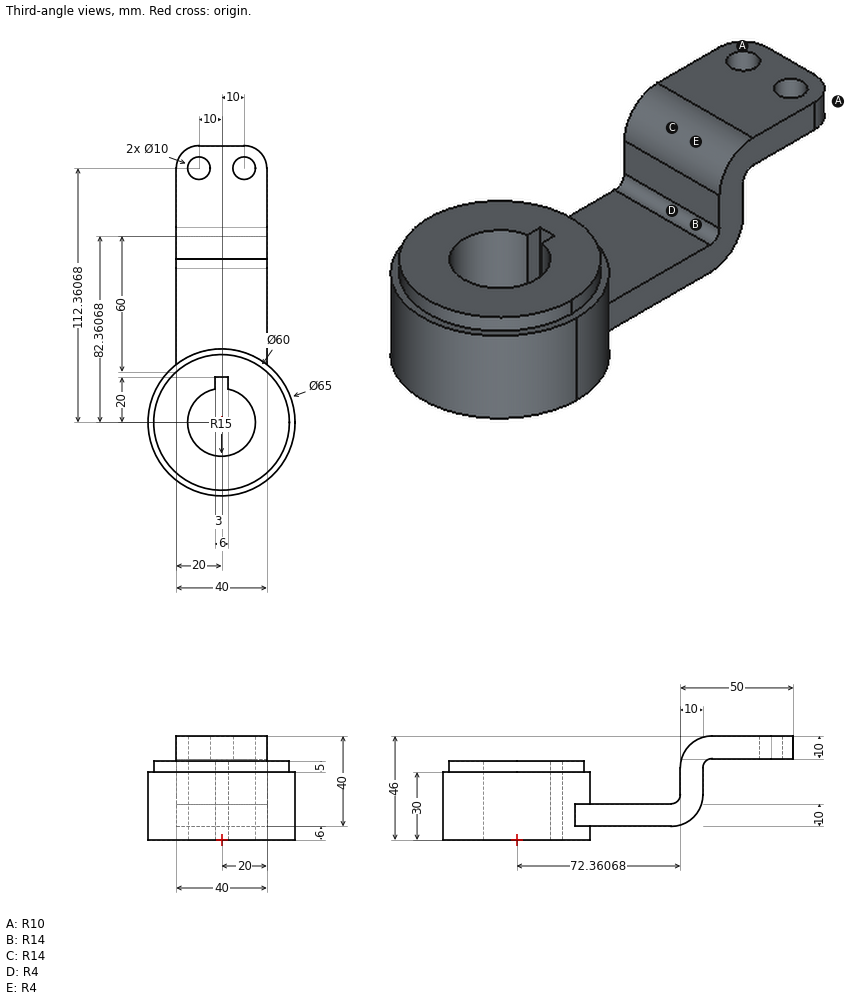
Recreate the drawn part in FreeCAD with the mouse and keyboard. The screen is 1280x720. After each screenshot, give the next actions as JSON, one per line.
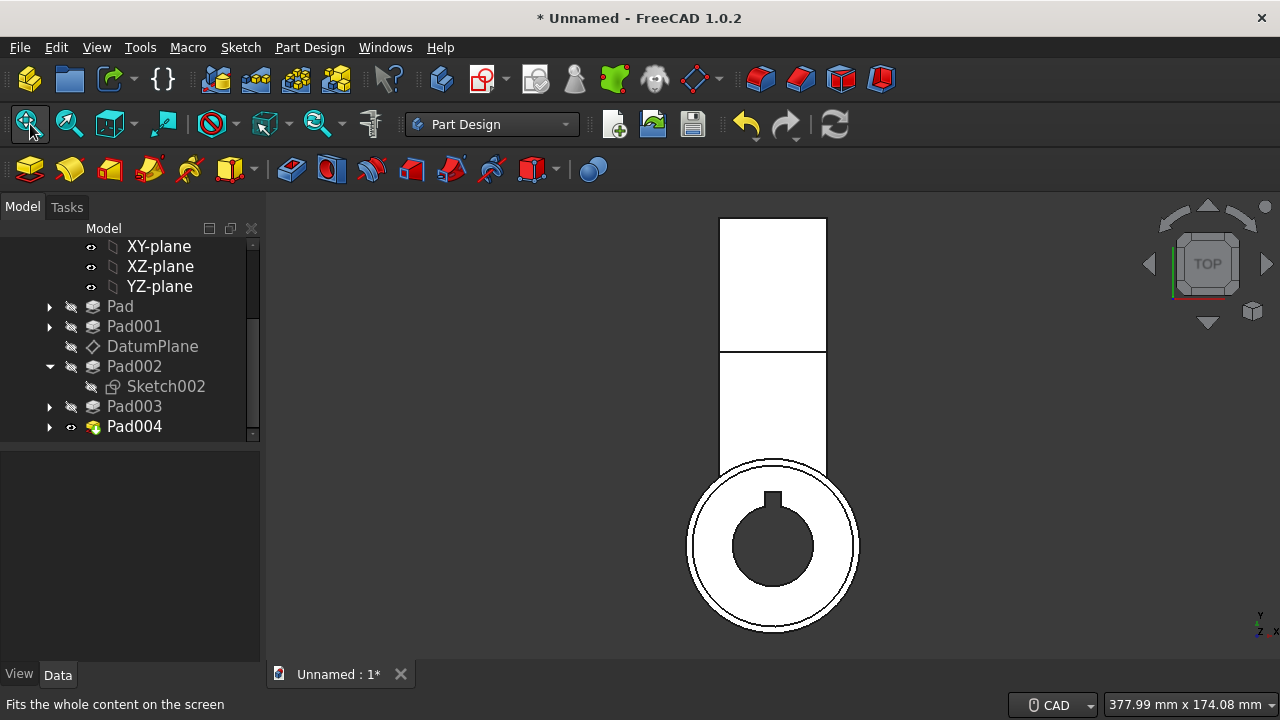
{"action": "key", "text": "0"}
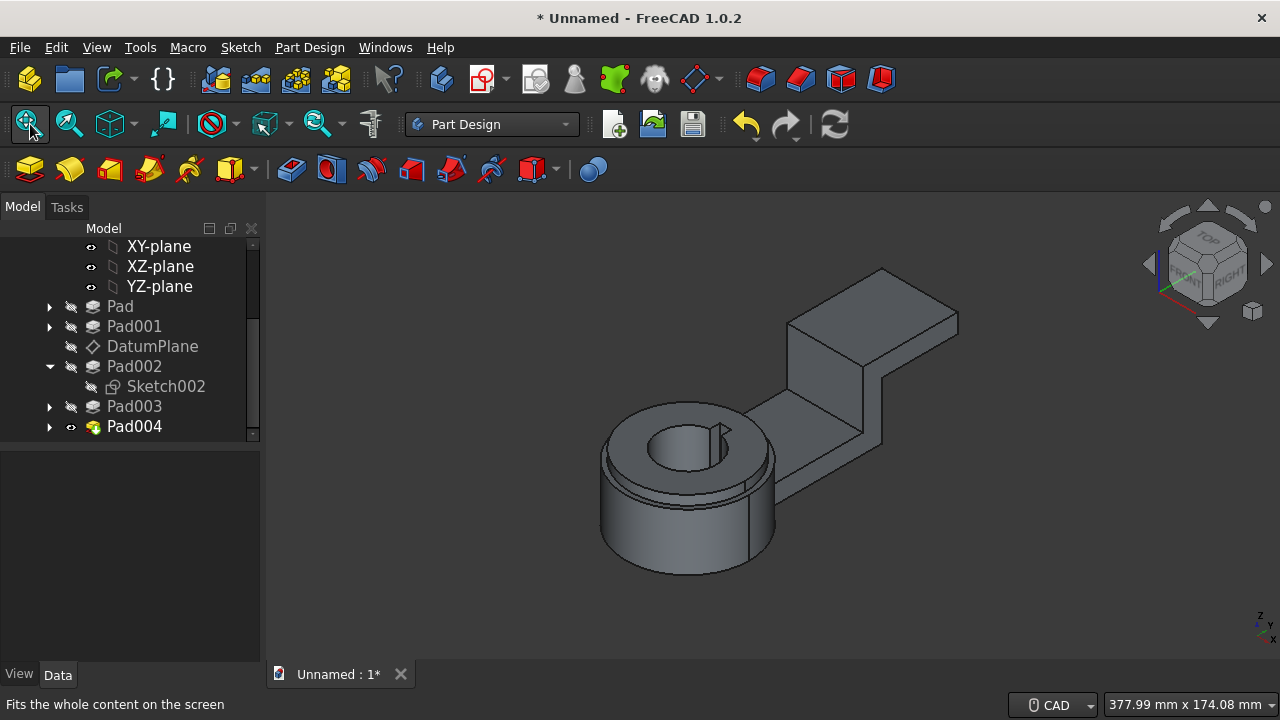
{"action": "key", "text": "1"}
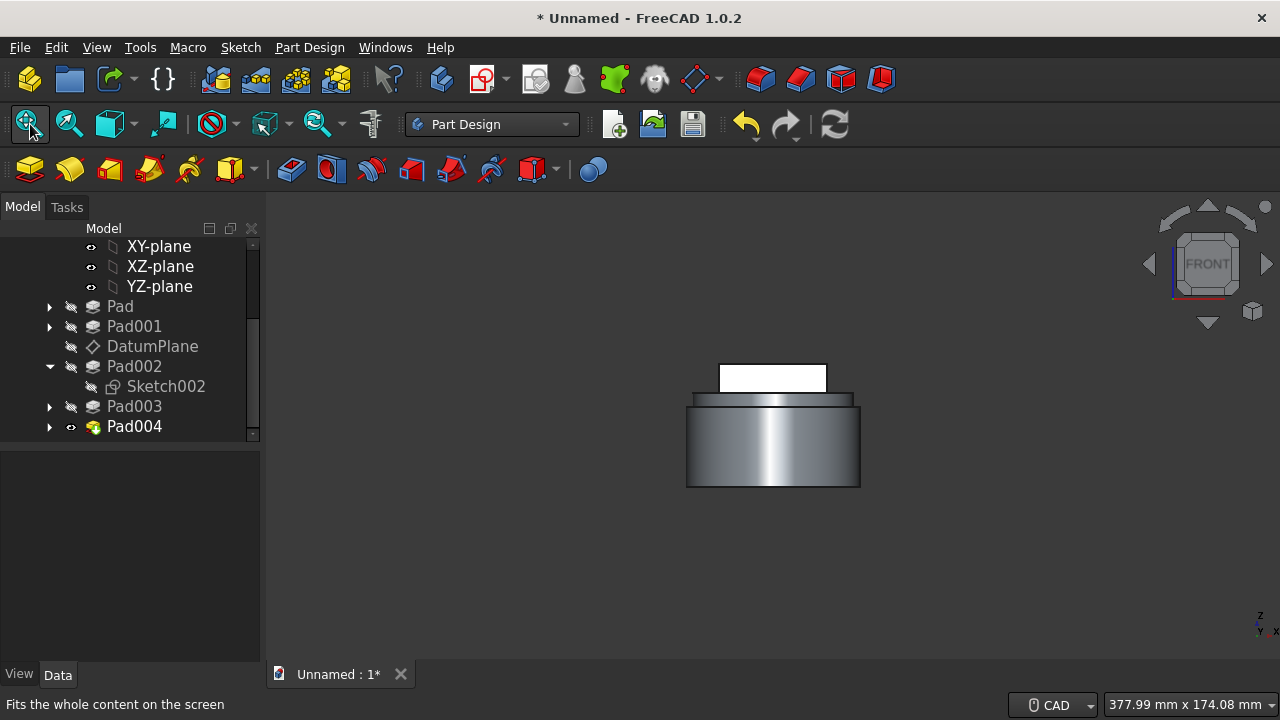
{"action": "key", "text": "v f"}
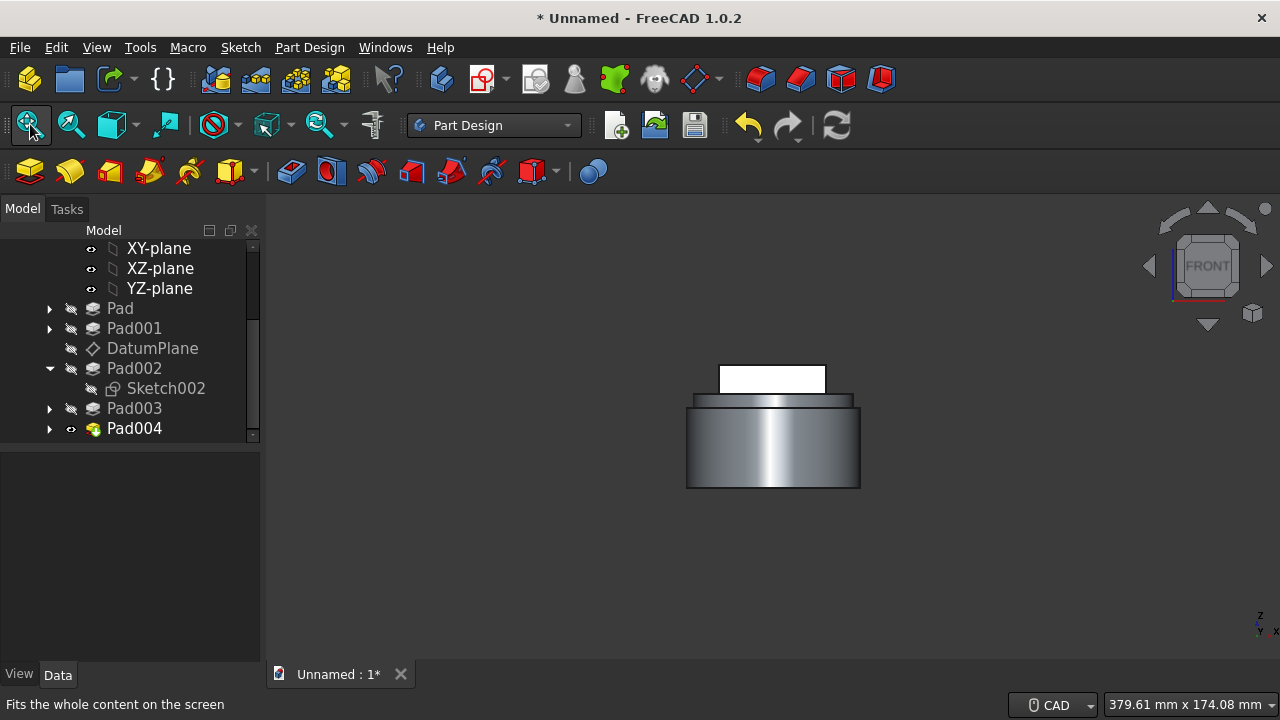
{"action": "key", "text": "3"}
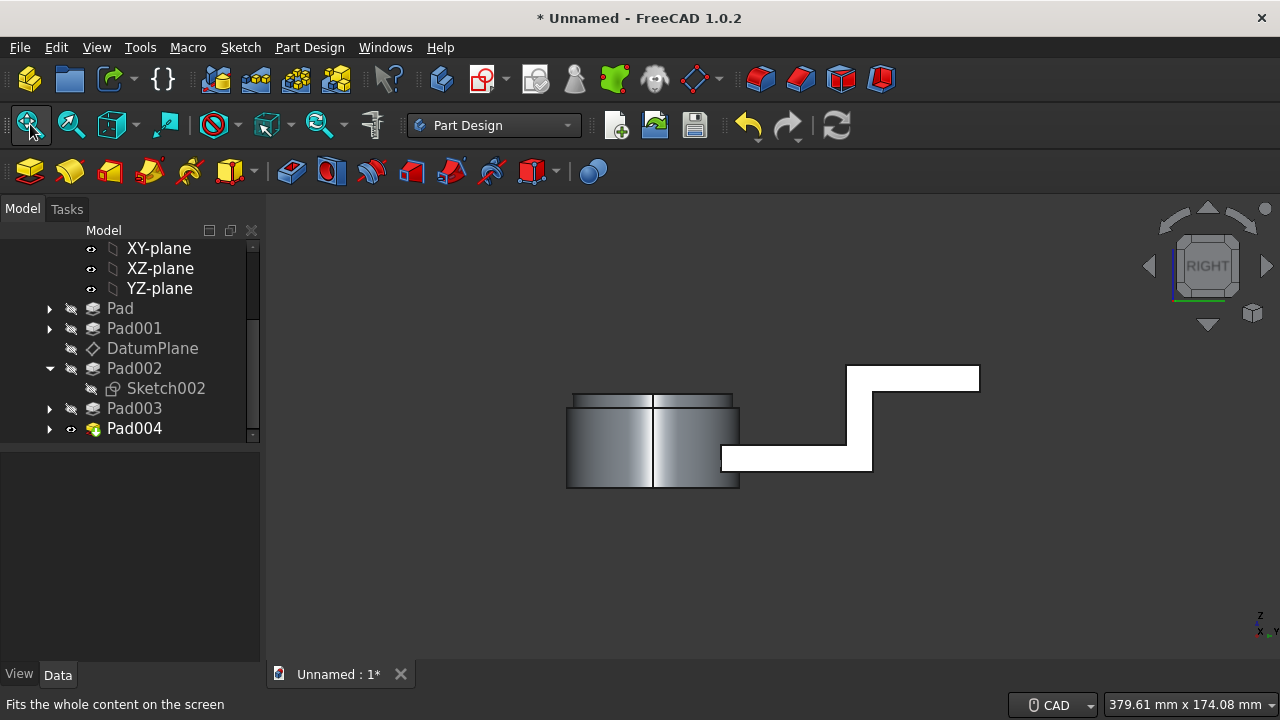
{"action": "key", "text": "v f"}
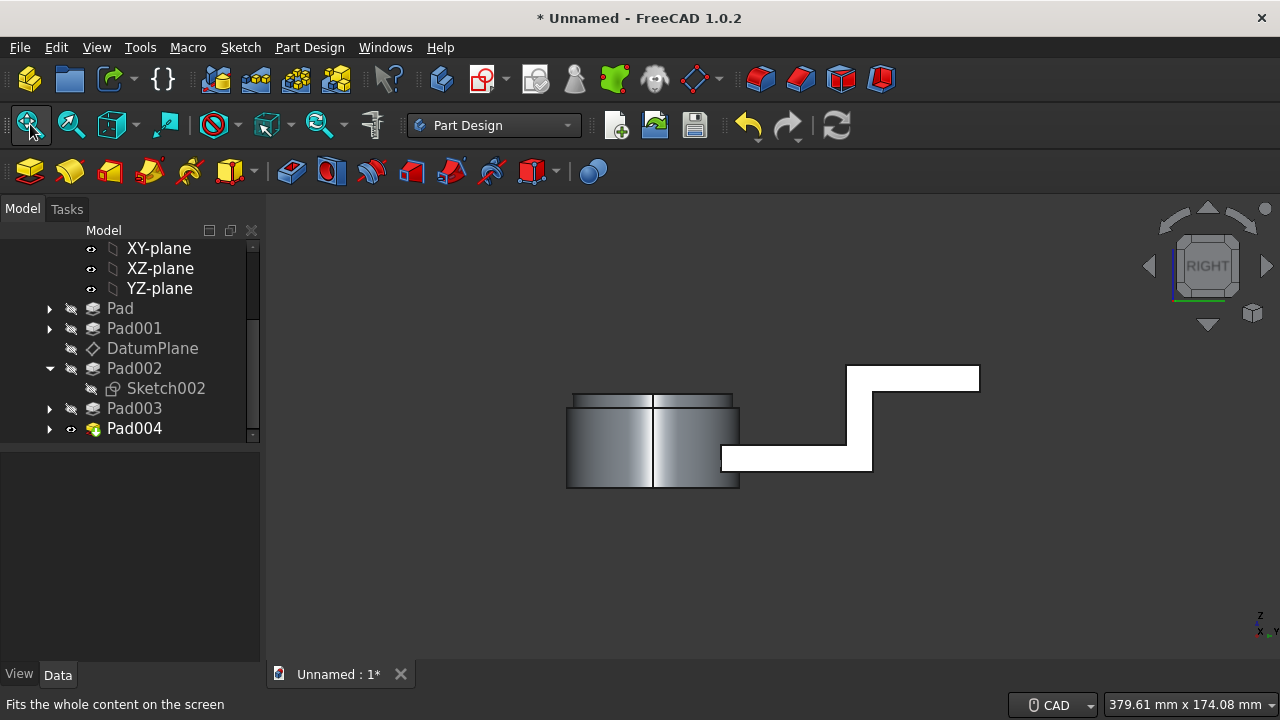
{"action": "left_click", "coordinate": [980, 377]}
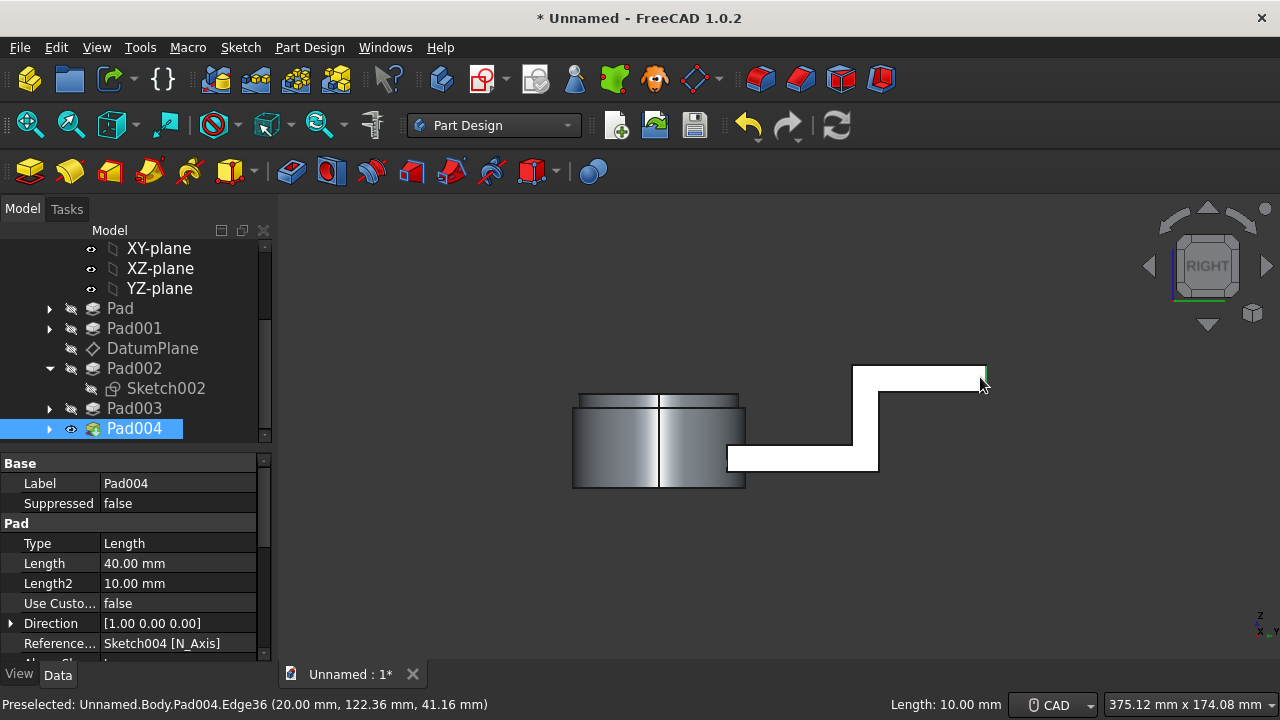
{"action": "key", "text": "5"}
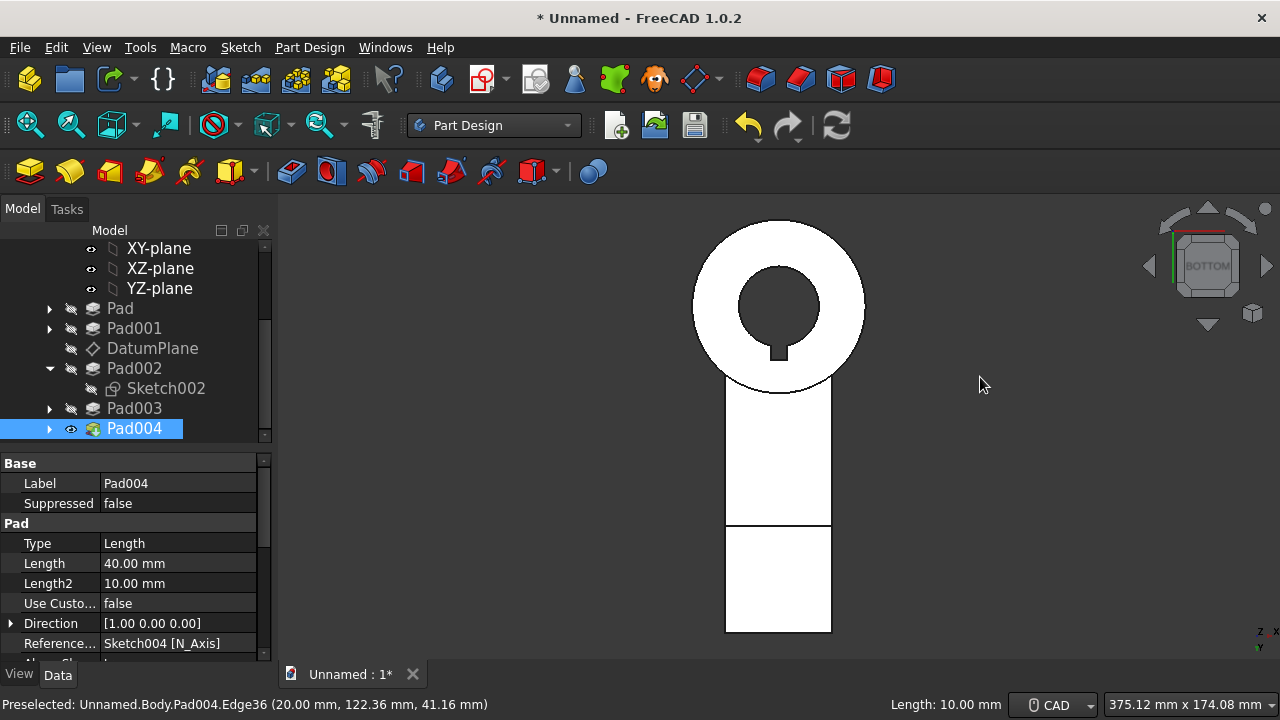
{"action": "key", "text": "4"}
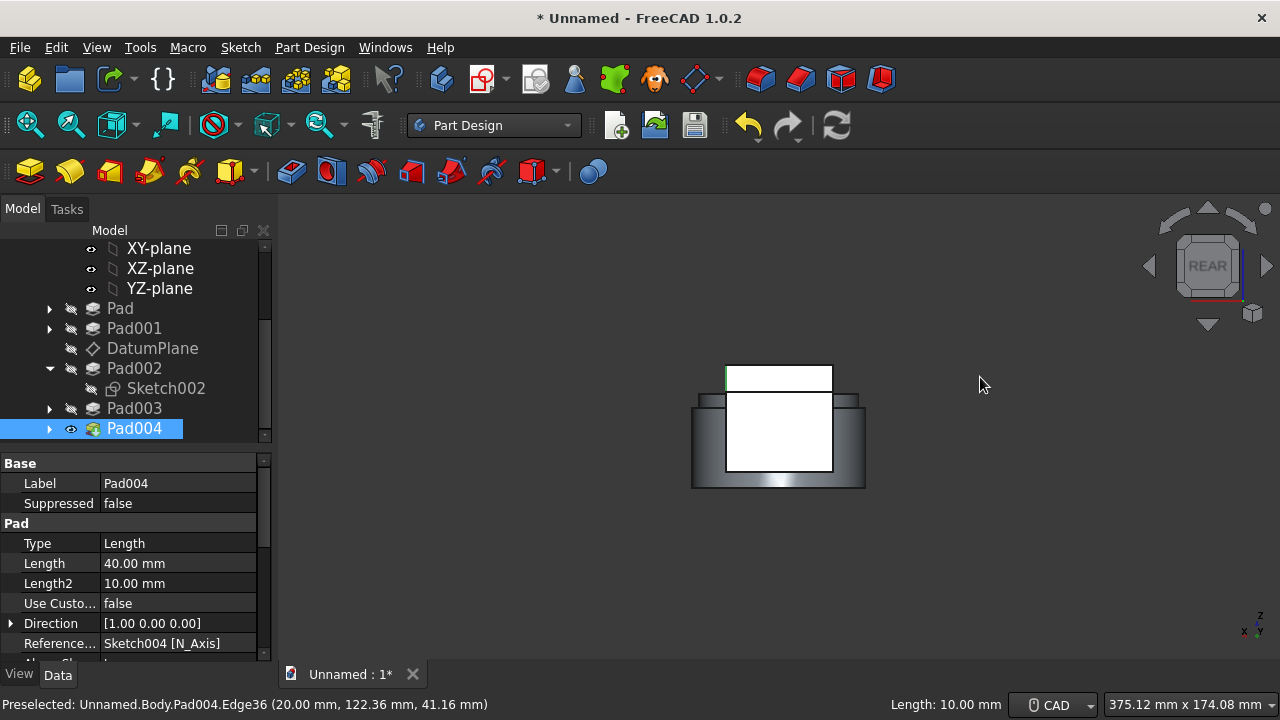
{"action": "left_click", "coordinate": [32, 126]}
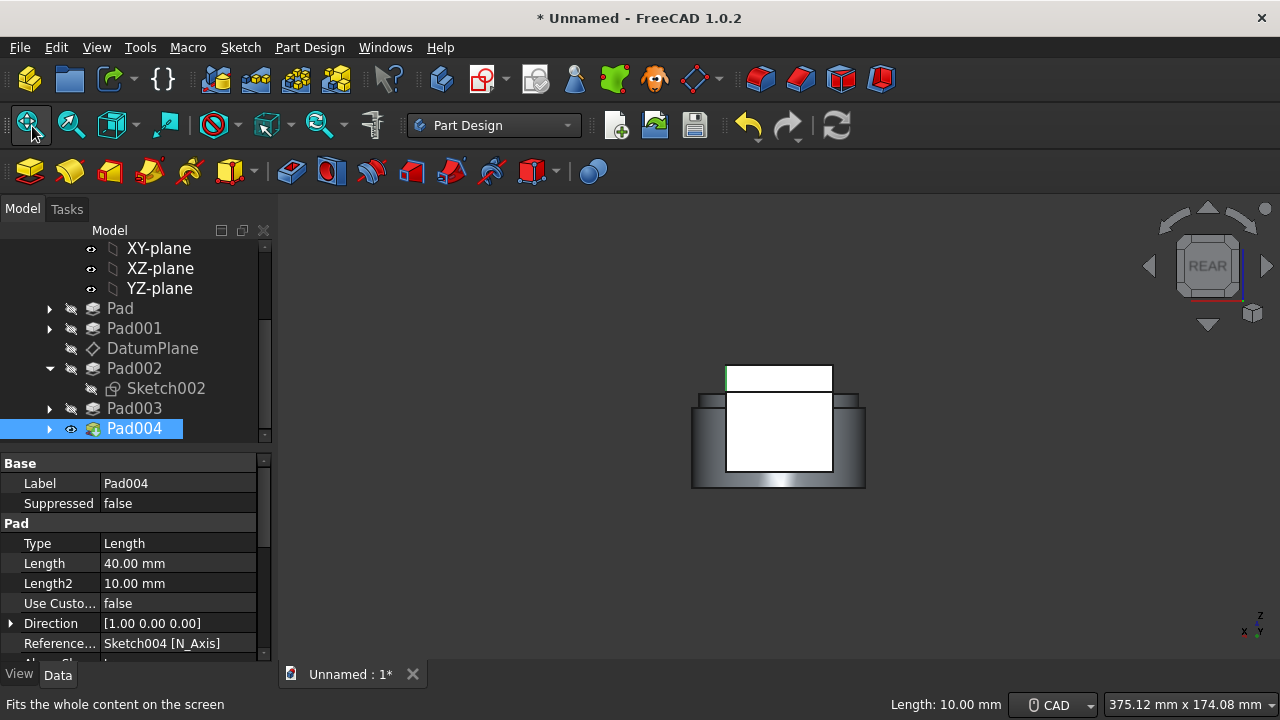
{"action": "left_click", "coordinate": [833, 377], "text": "ctrl"}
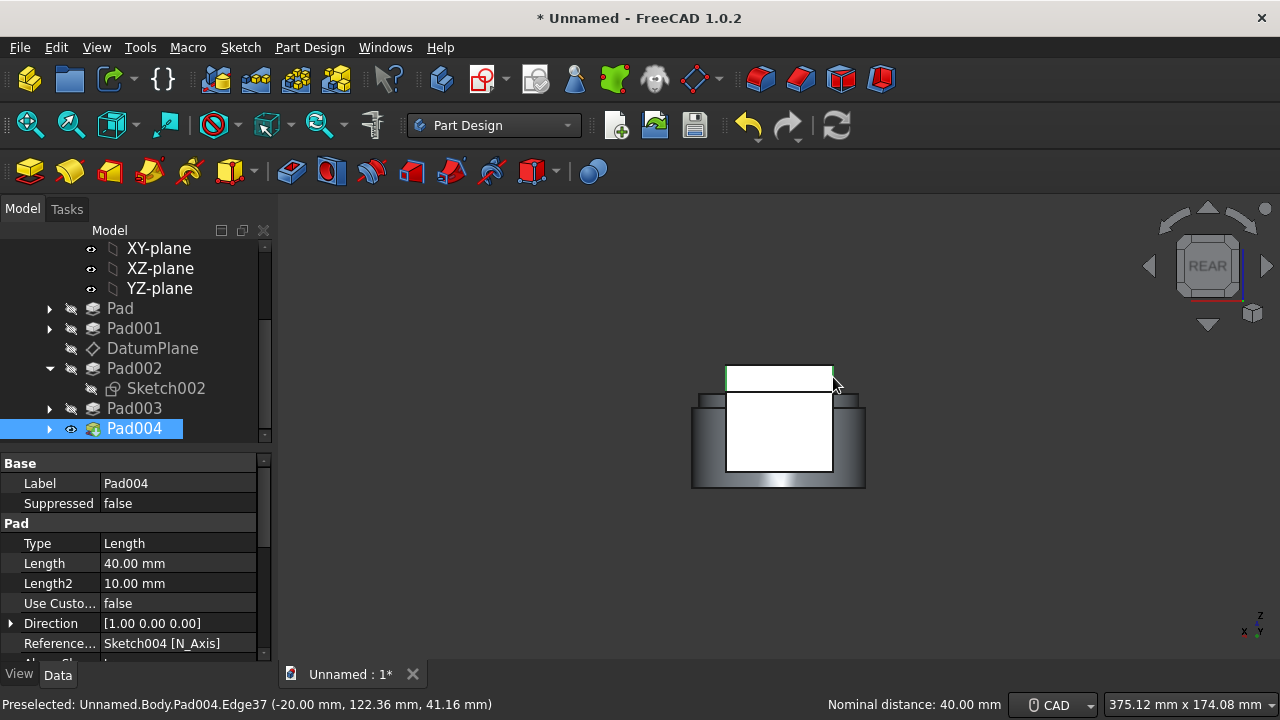
{"action": "left_click", "coordinate": [762, 80]}